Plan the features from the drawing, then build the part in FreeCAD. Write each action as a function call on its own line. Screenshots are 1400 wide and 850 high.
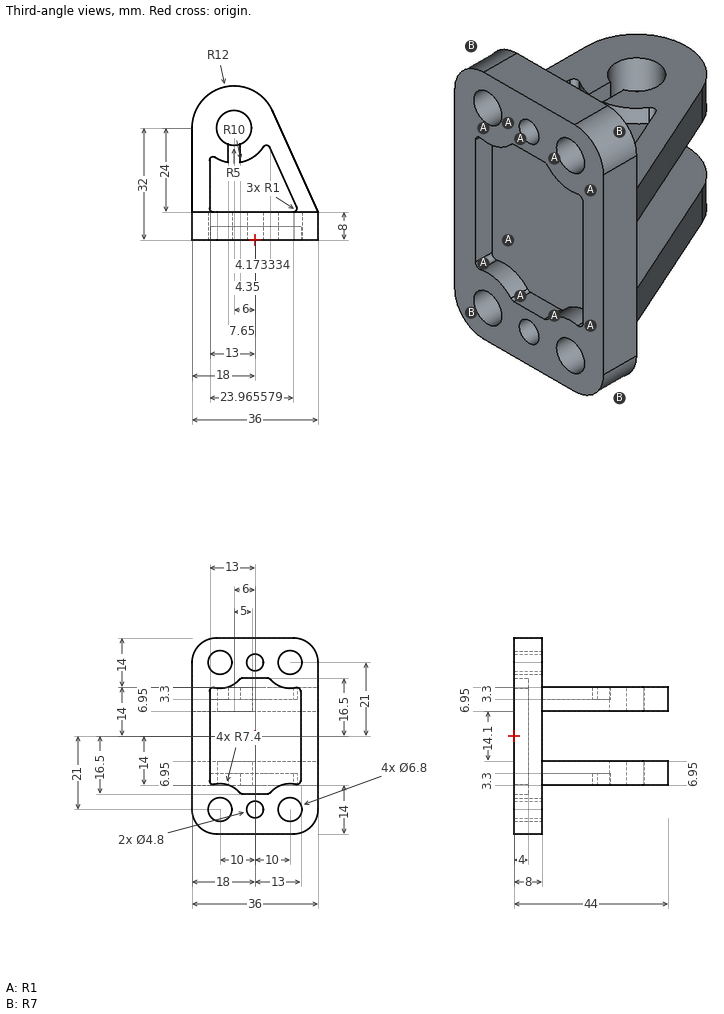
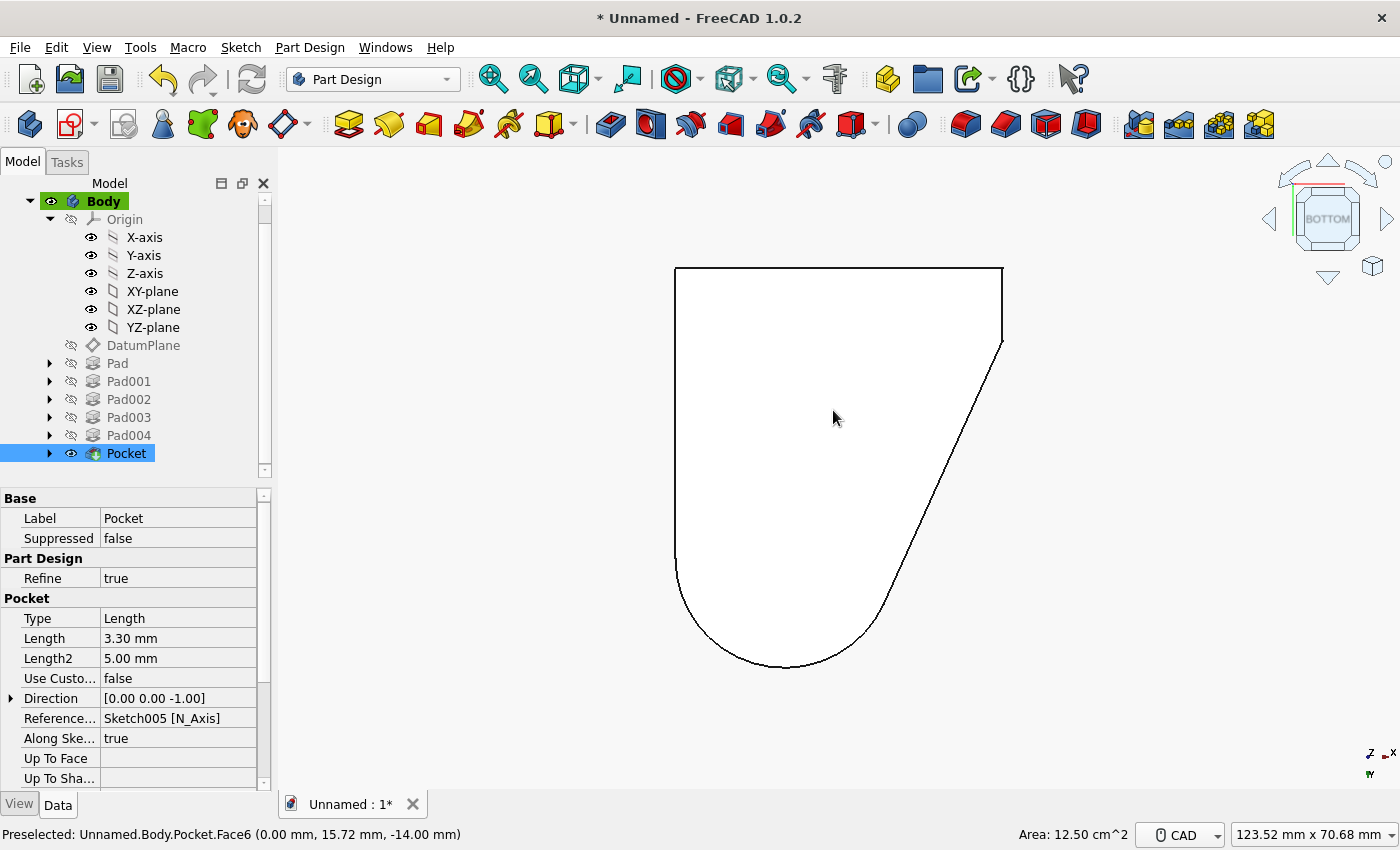
click(70, 124)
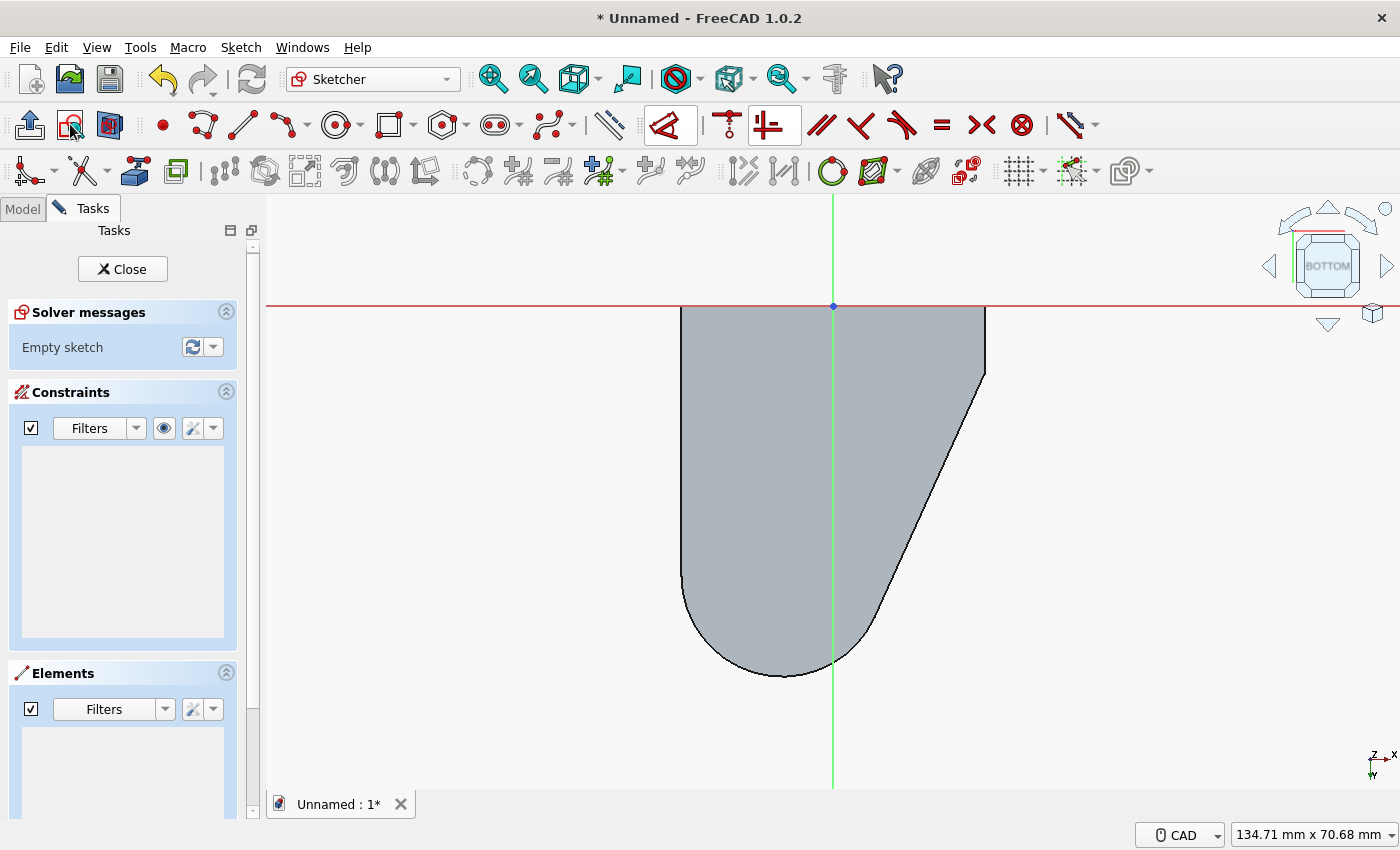
scroll(889, 222, up, 4)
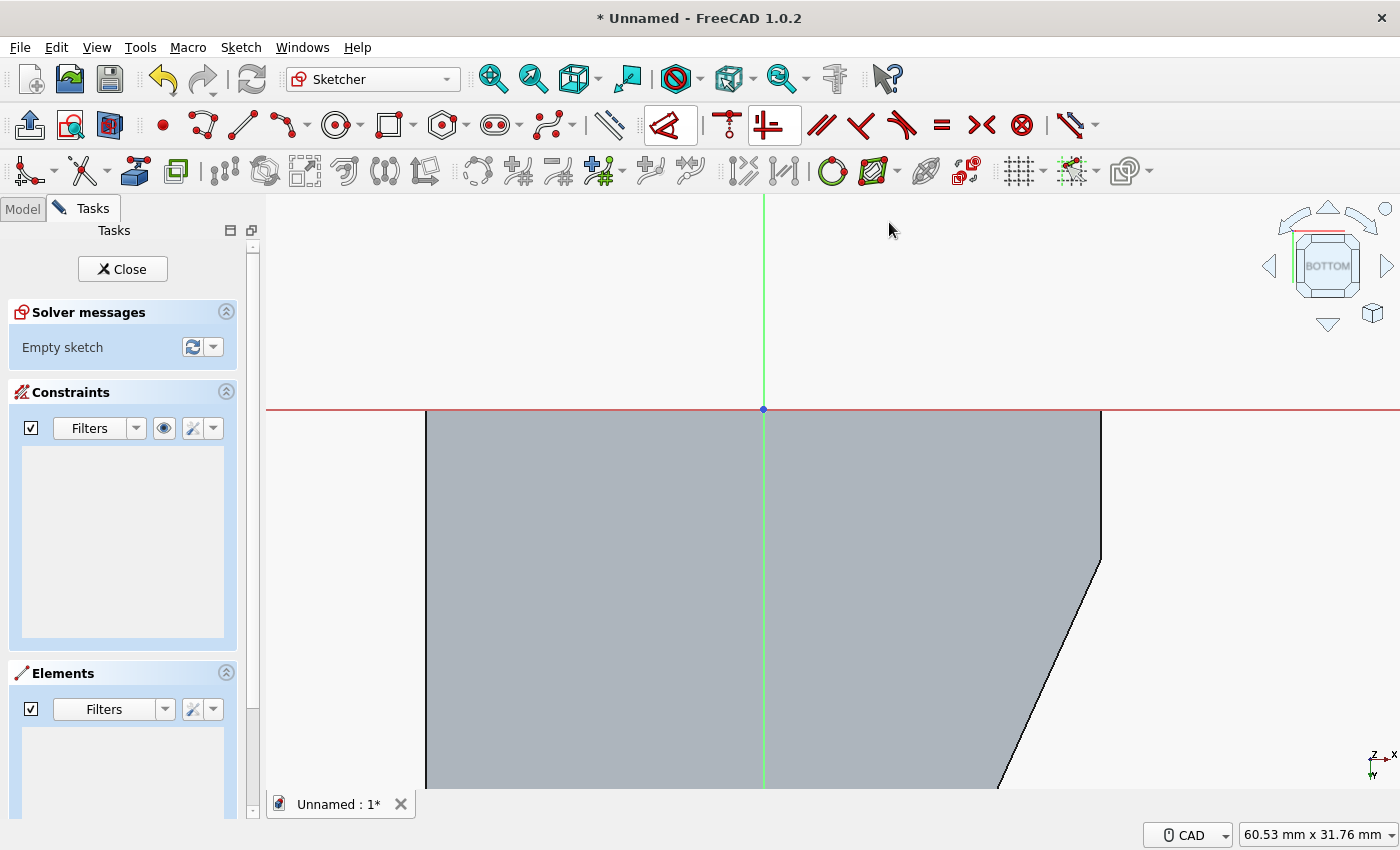
key(g)
key(r)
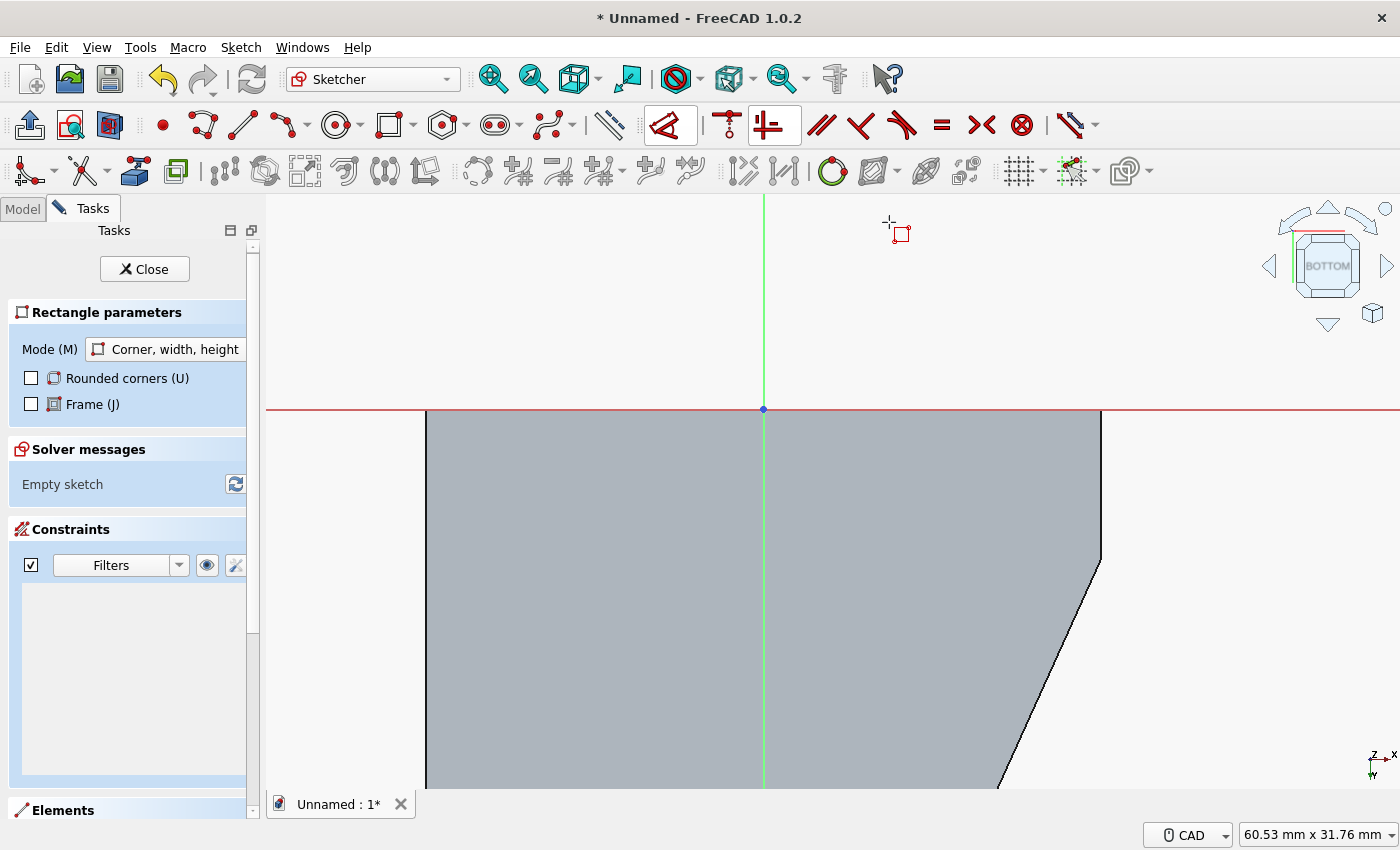
click(426, 410)
move(1101, 559)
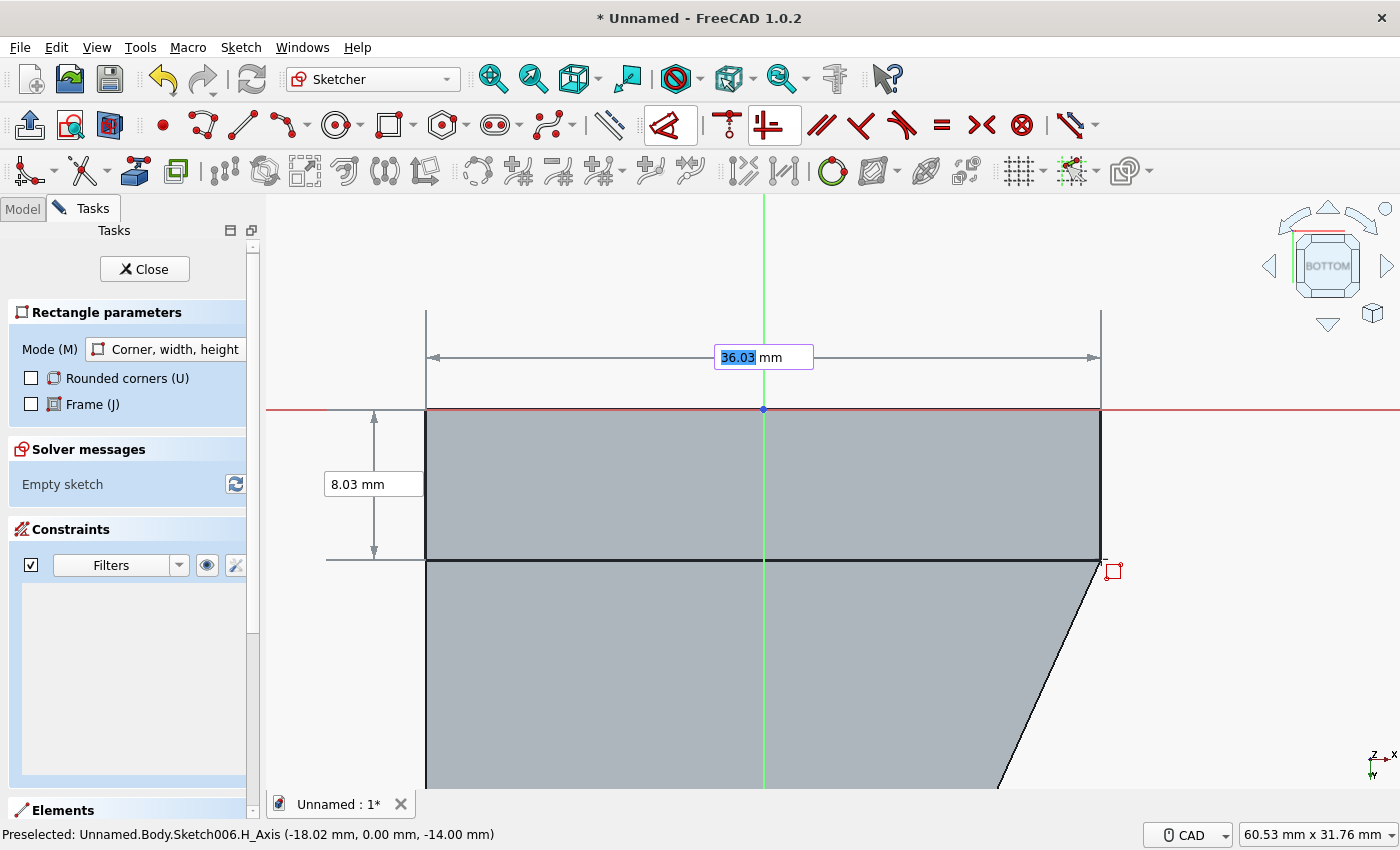
text(36)
key(Tab)
text(8)
key(Return)
key(Escape)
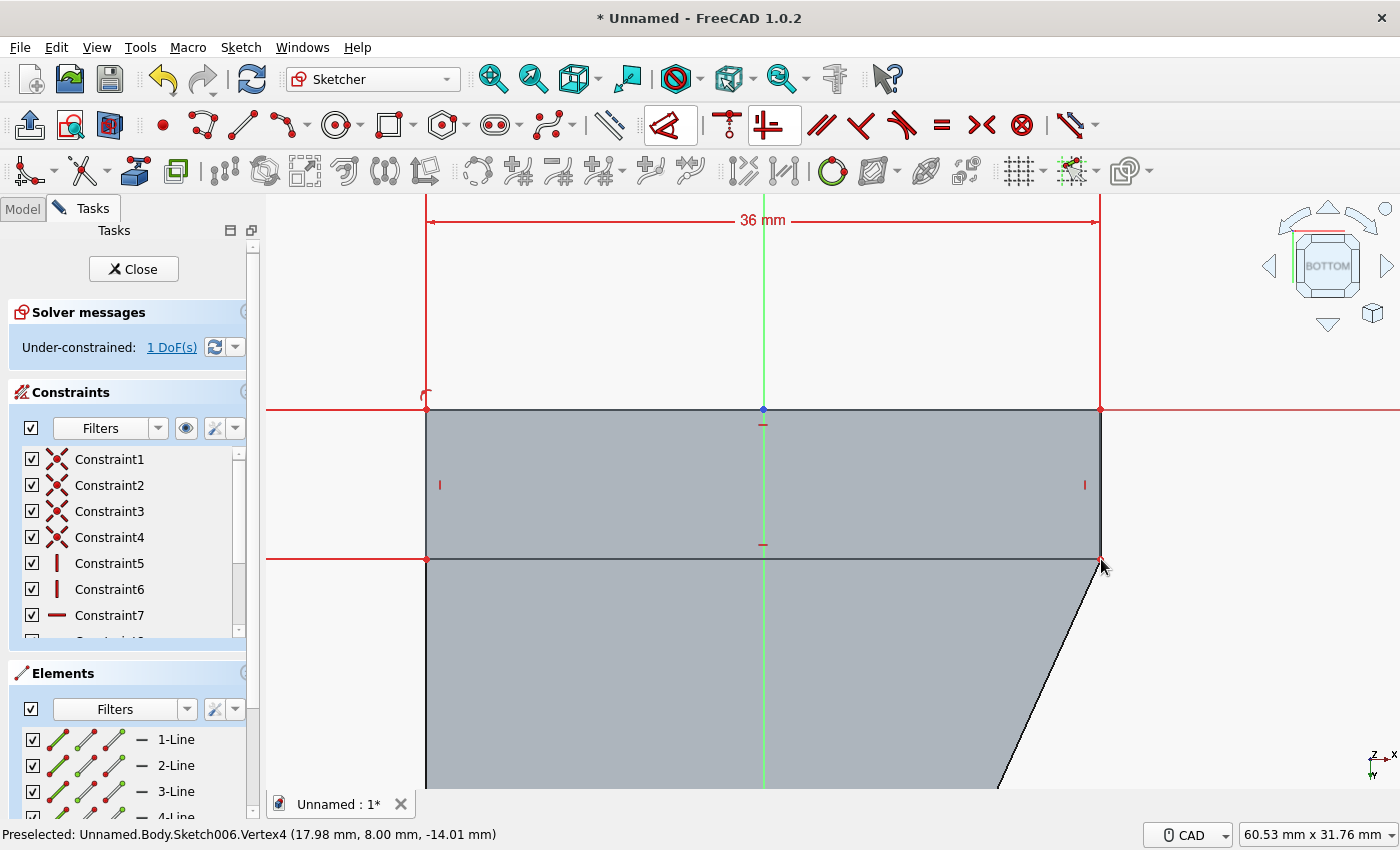
click(426, 410)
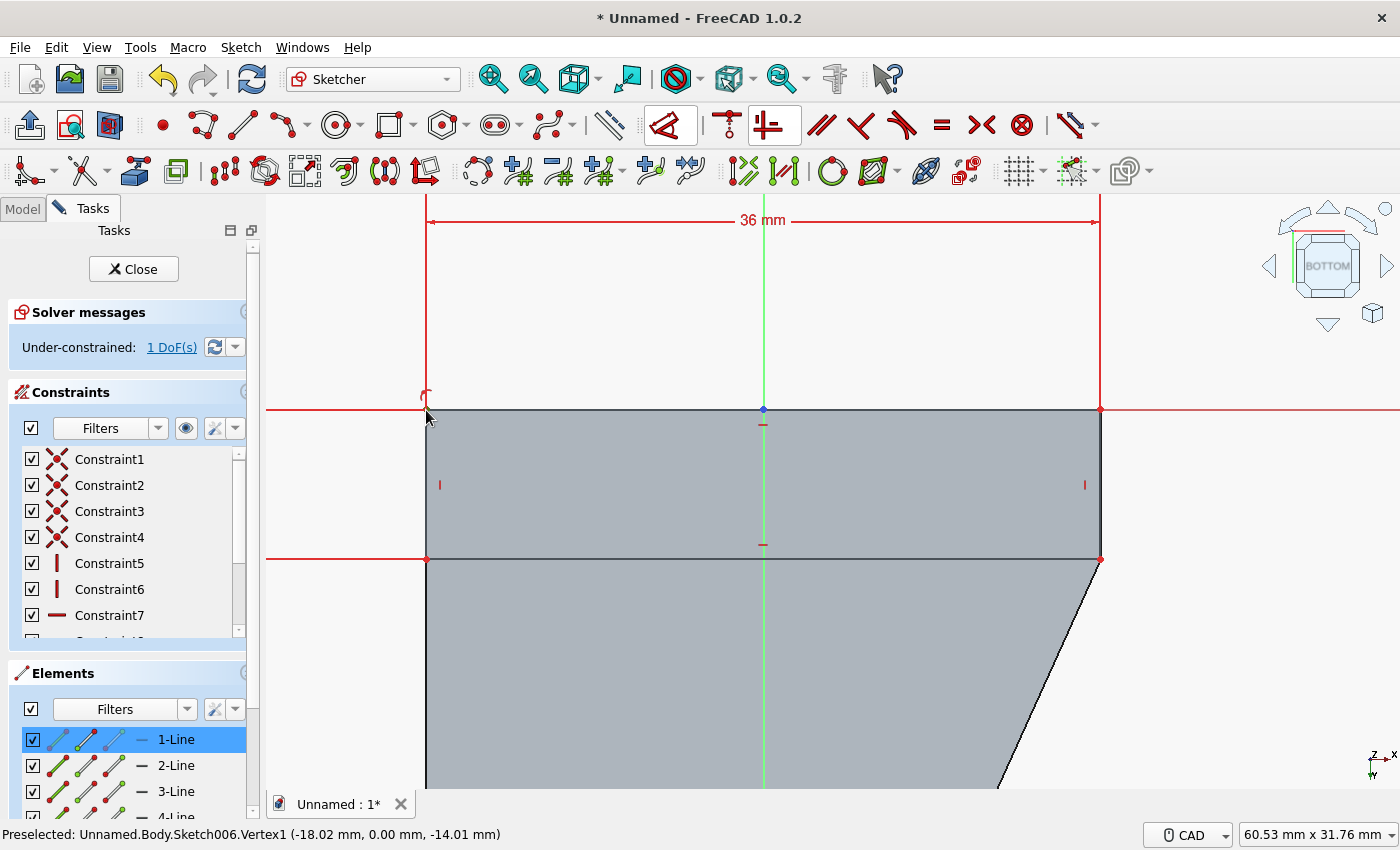
click(692, 126)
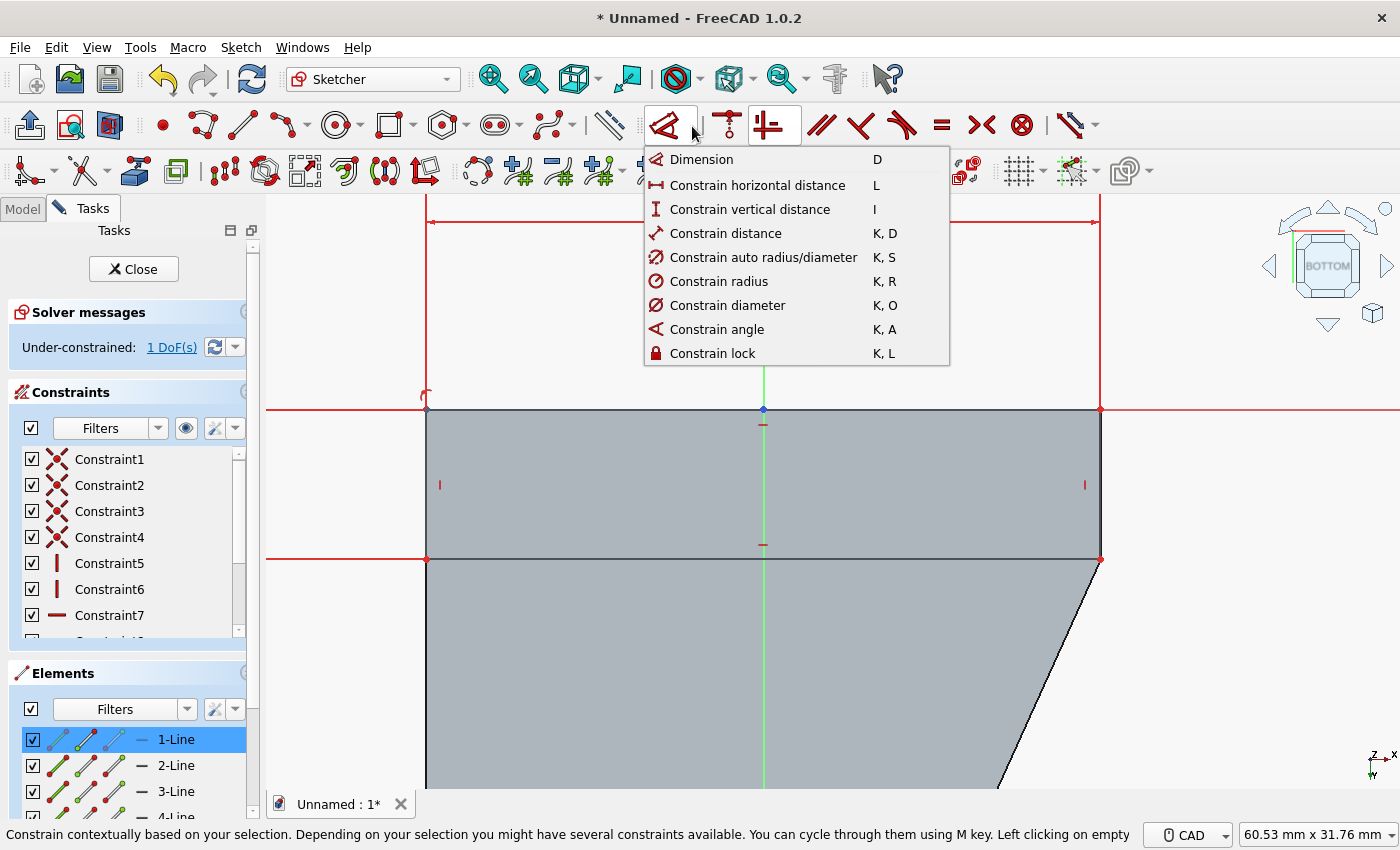
click(797, 185)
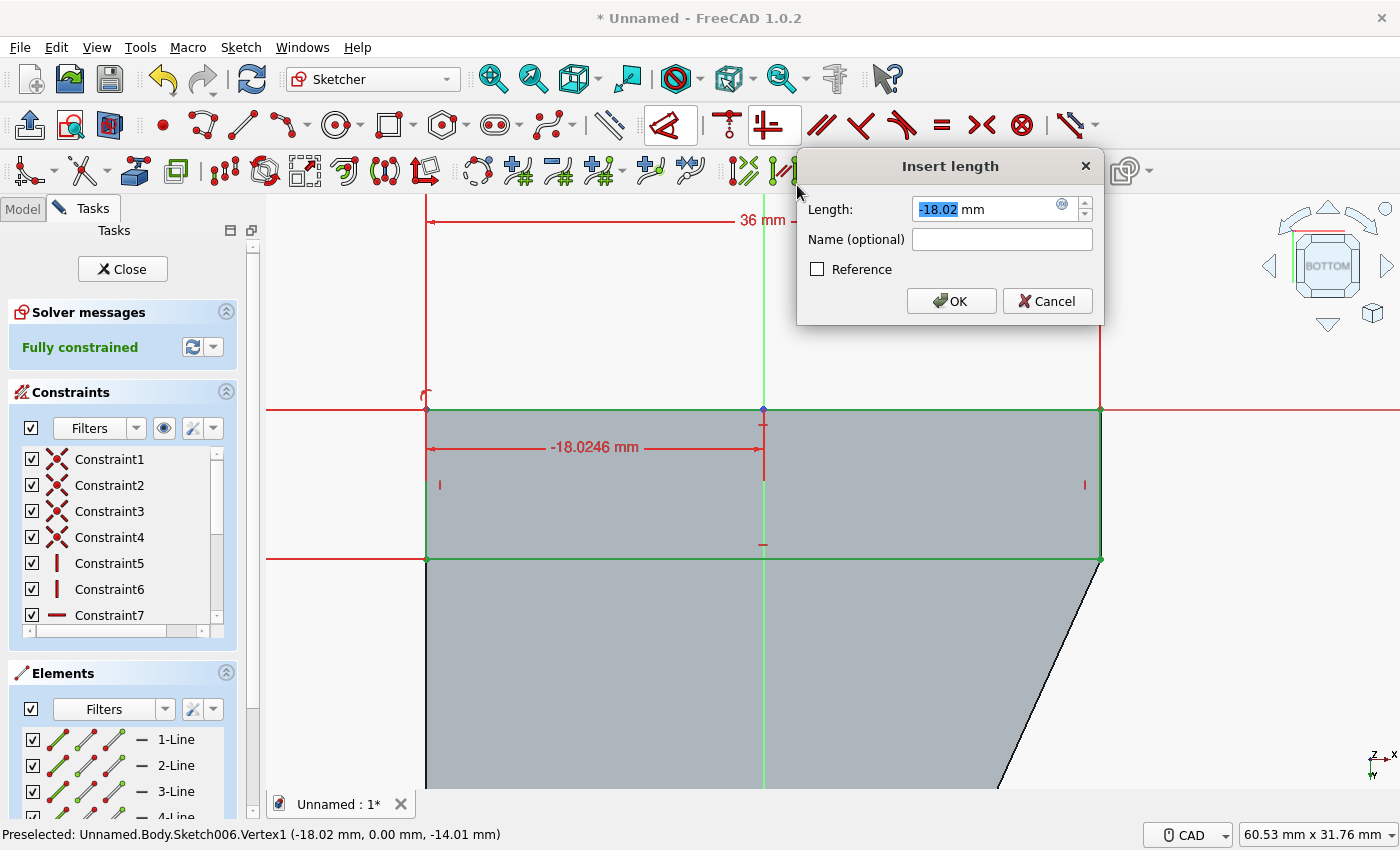
text(-18)
key(Return)